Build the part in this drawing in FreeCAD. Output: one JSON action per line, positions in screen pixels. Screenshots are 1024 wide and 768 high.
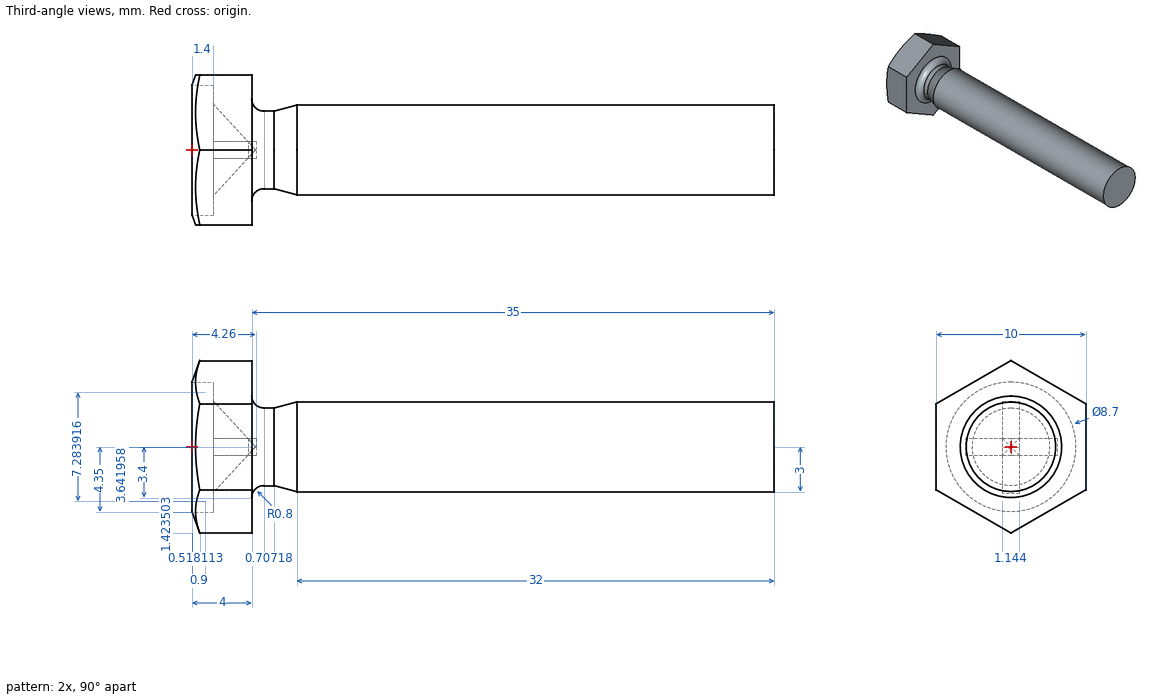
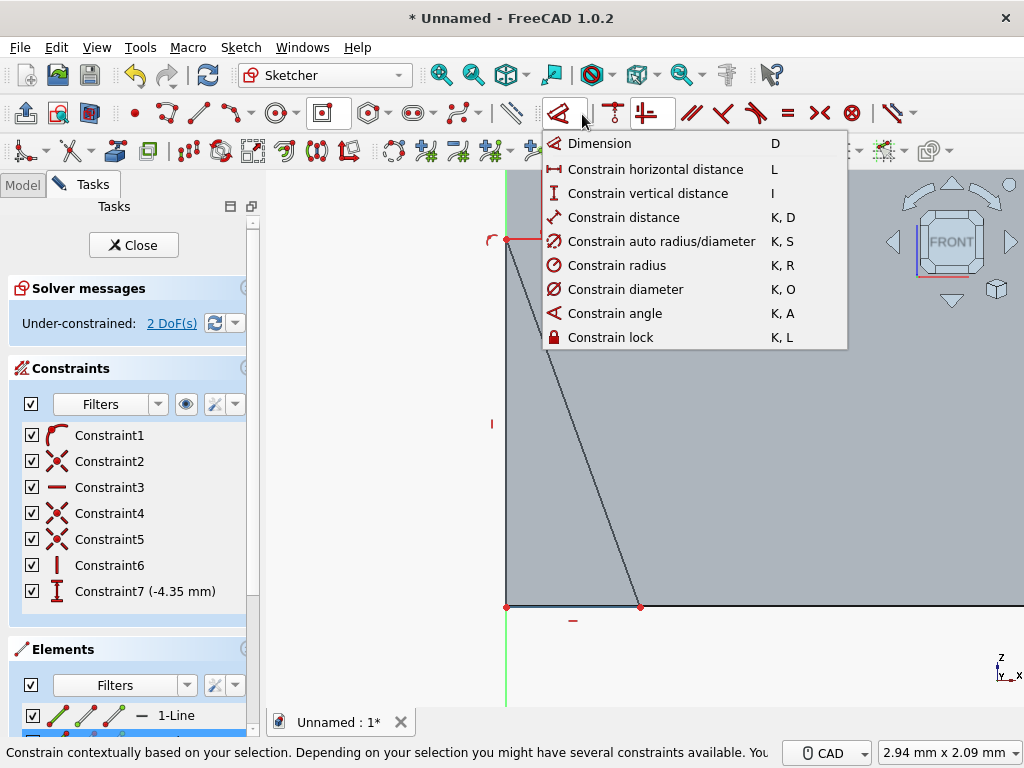
{"action": "left_click", "coordinate": [695, 169]}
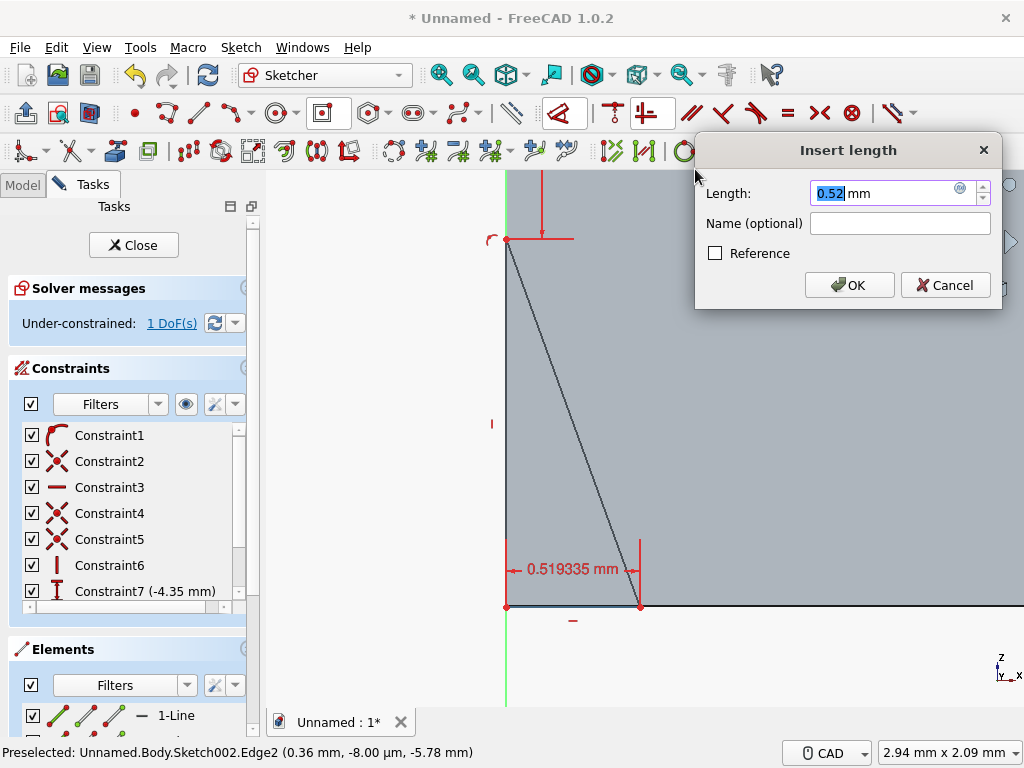
{"action": "type", "text": "0.518113"}
{"action": "key", "text": "Return"}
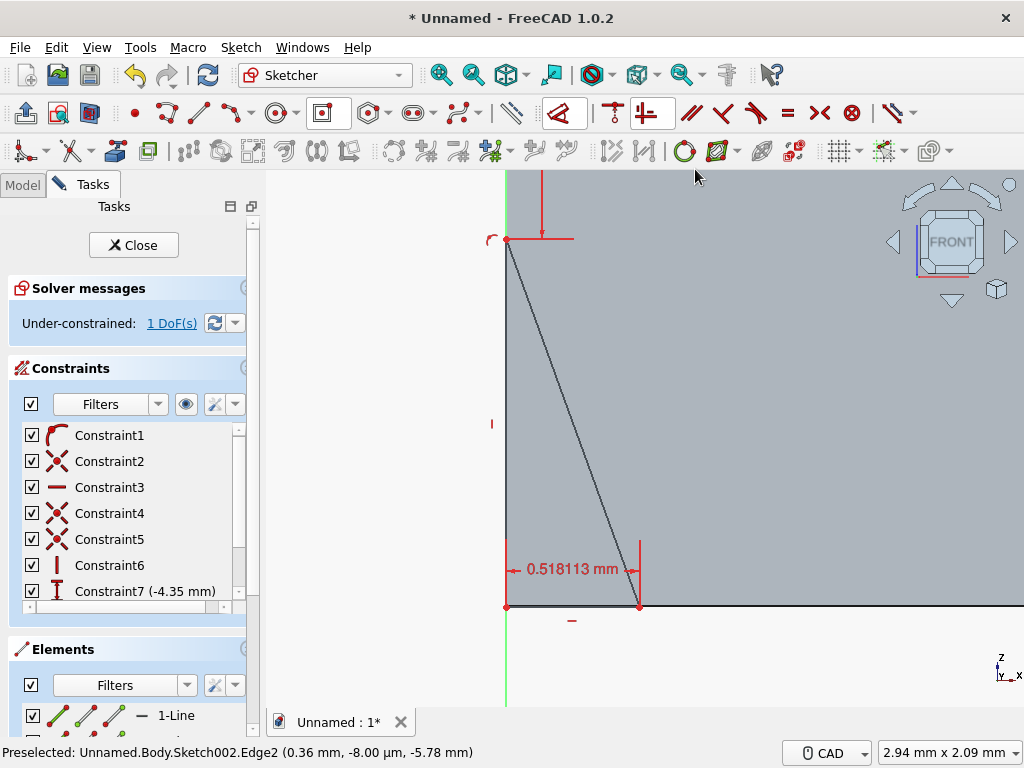
{"action": "left_click", "coordinate": [506, 497]}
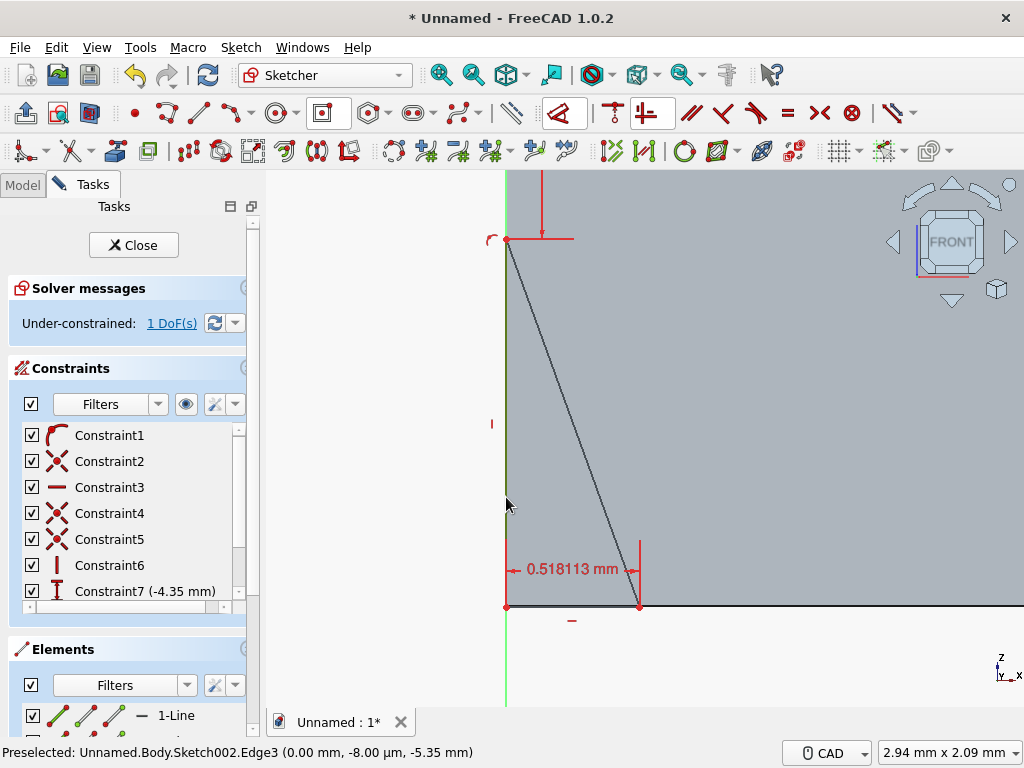
{"action": "left_click", "coordinate": [582, 114]}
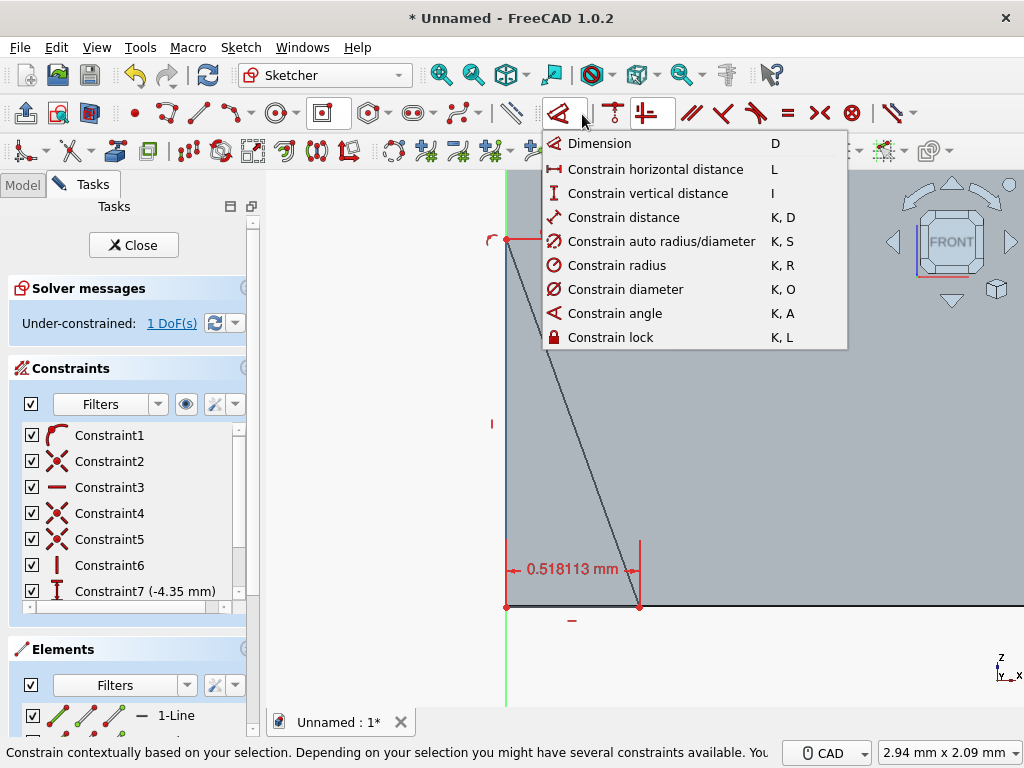
{"action": "left_click", "coordinate": [695, 193]}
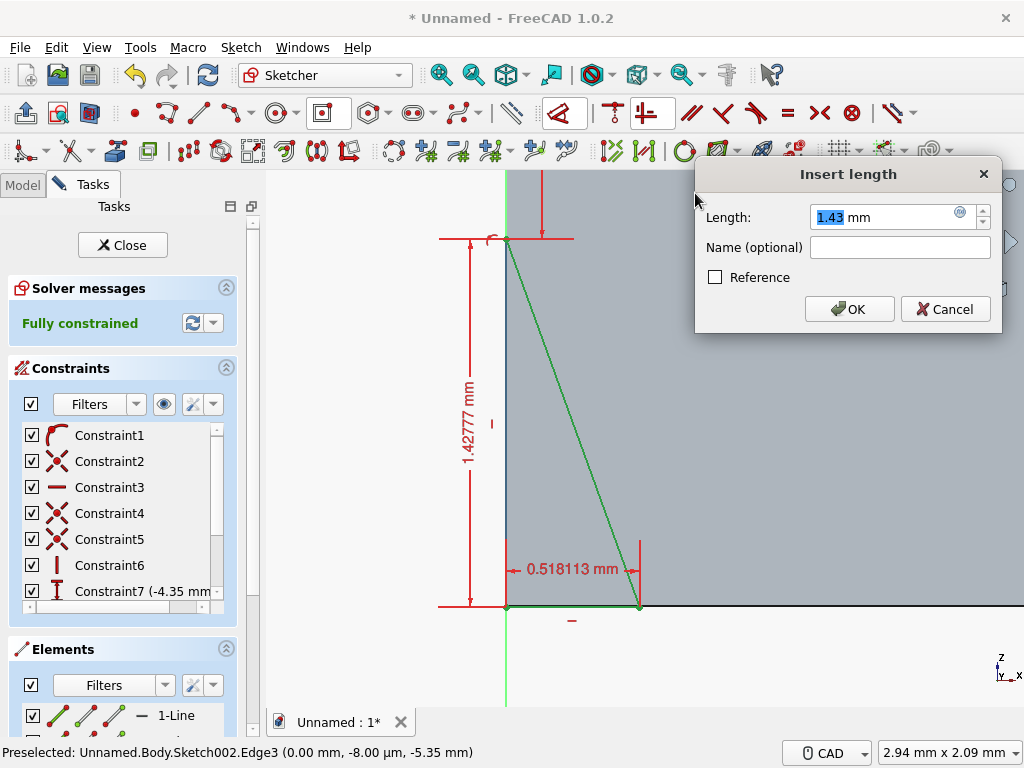
{"action": "type", "text": "1.423503"}
{"action": "key", "text": "Return"}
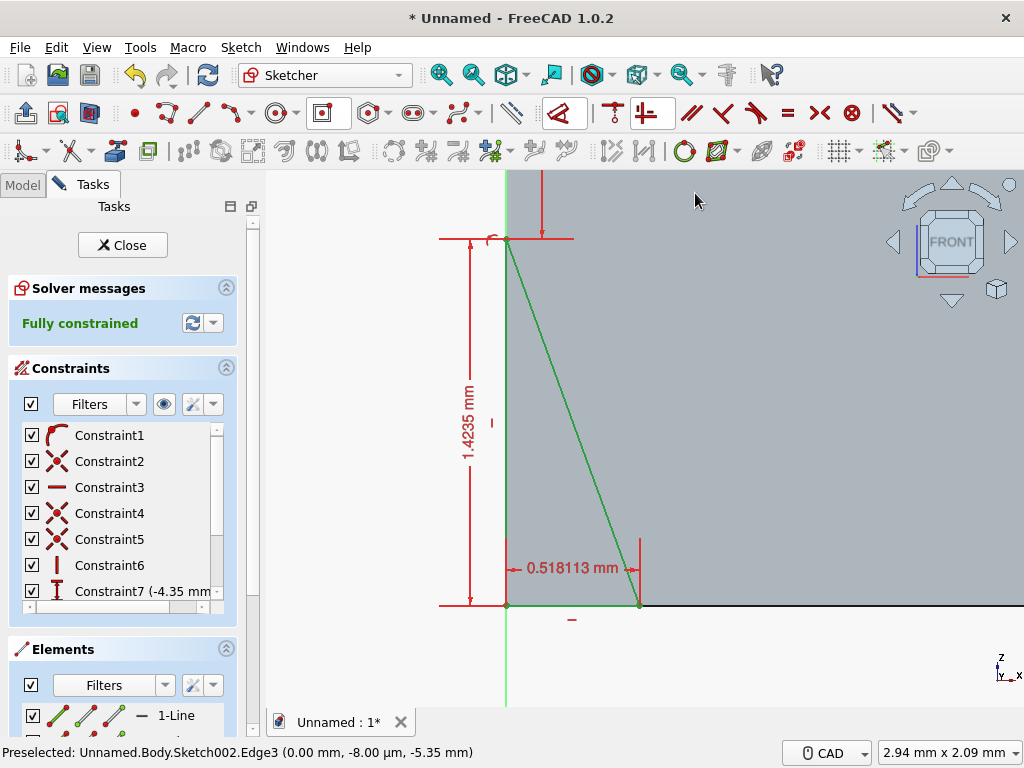
{"action": "left_click", "coordinate": [123, 245]}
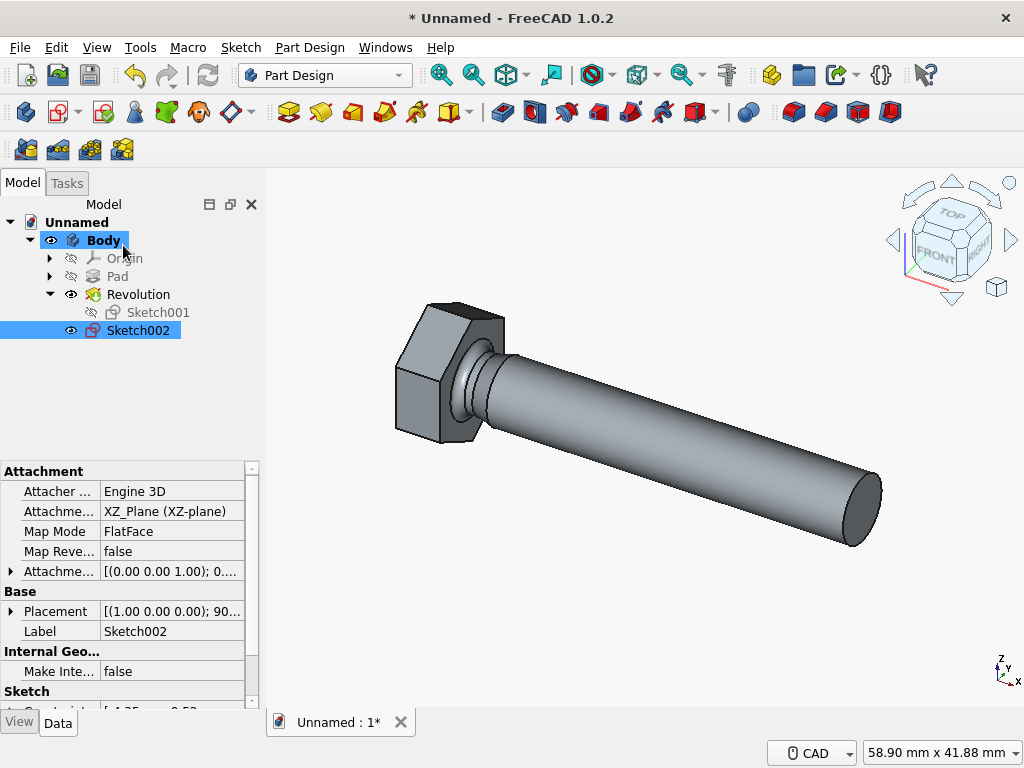
{"action": "left_click", "coordinate": [568, 112]}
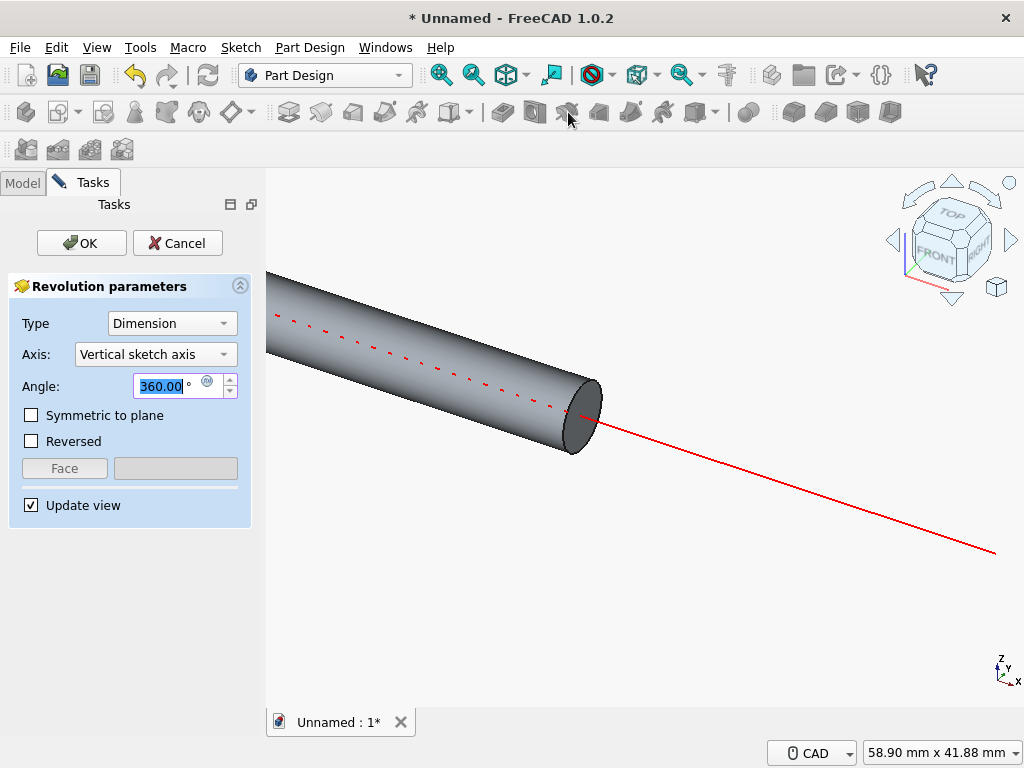
{"action": "left_click", "coordinate": [156, 354]}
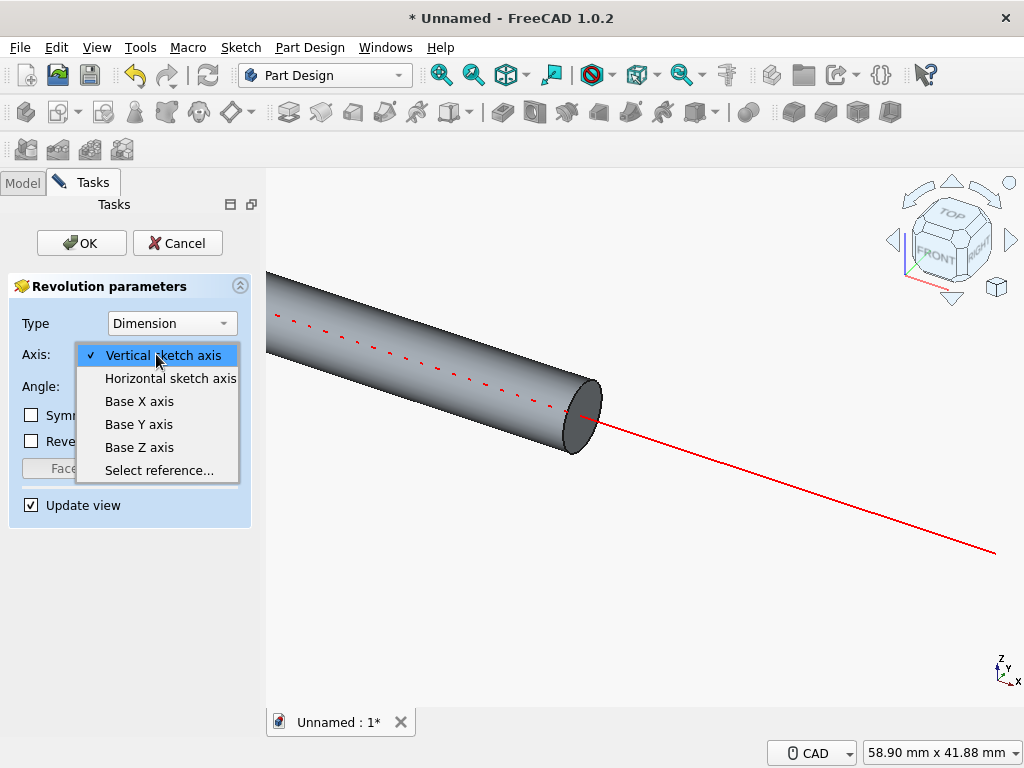
{"action": "left_click", "coordinate": [156, 378]}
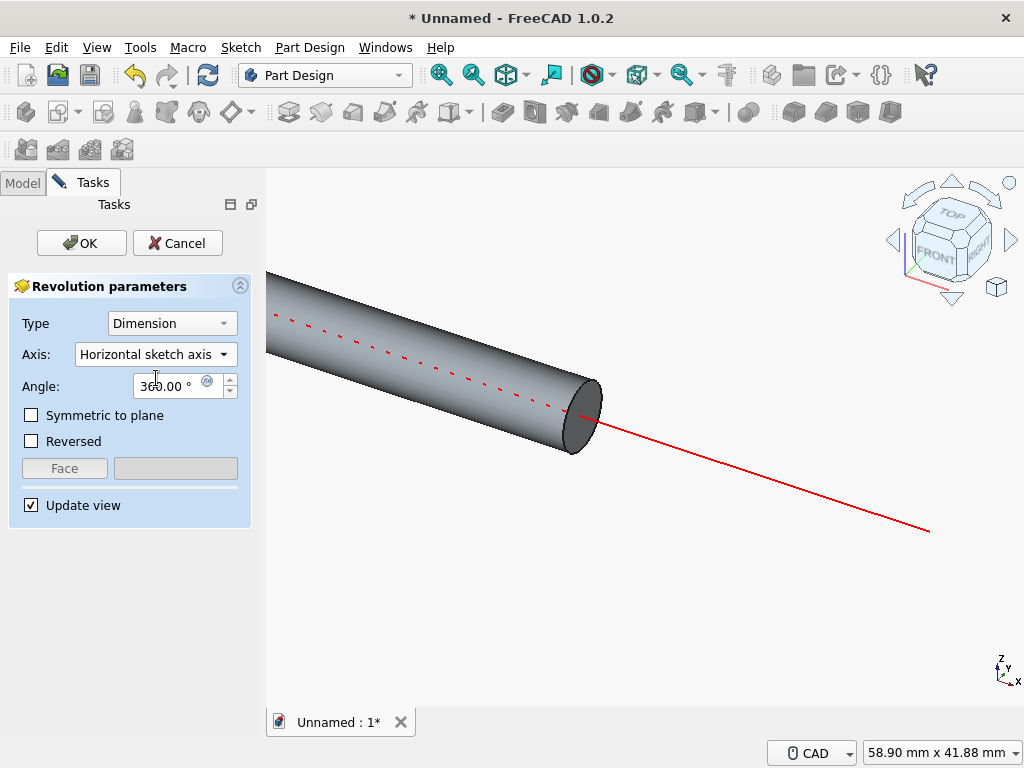
{"action": "left_click", "coordinate": [82, 243]}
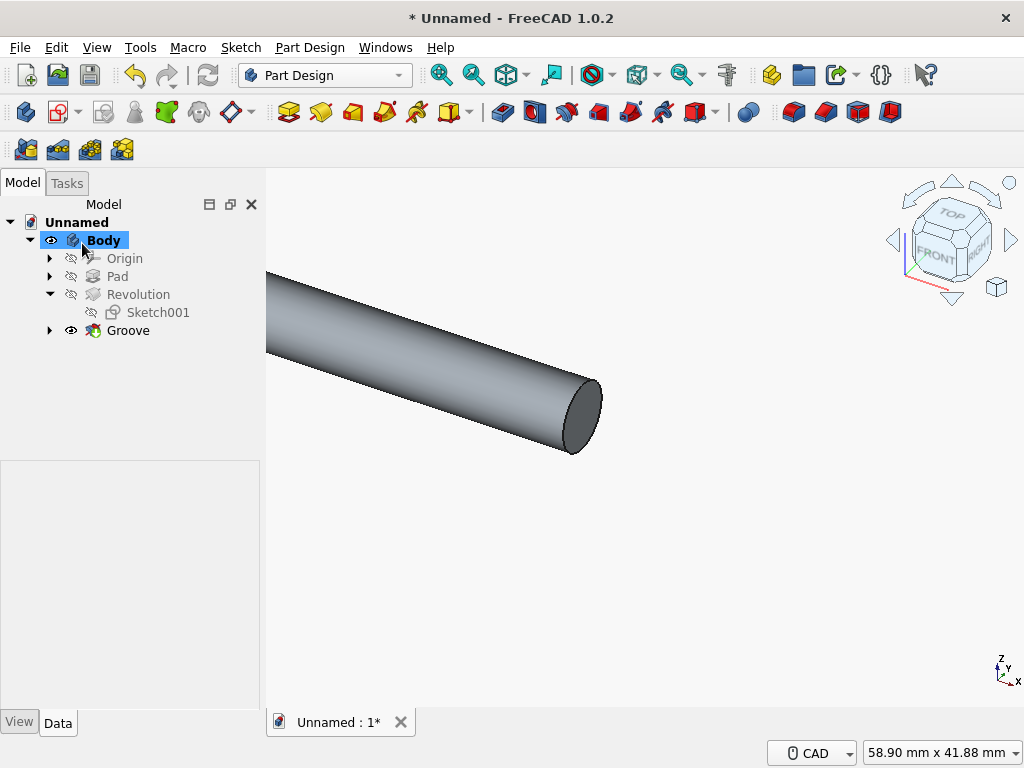
{"action": "left_click", "coordinate": [442, 76]}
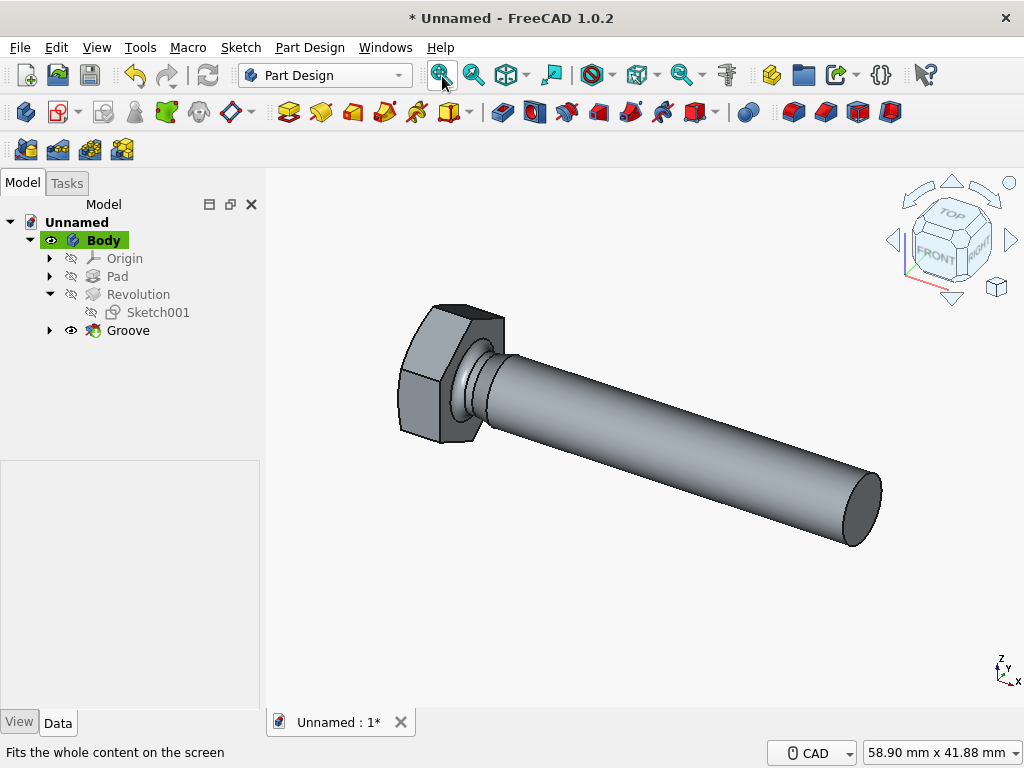
{"action": "key", "text": "6"}